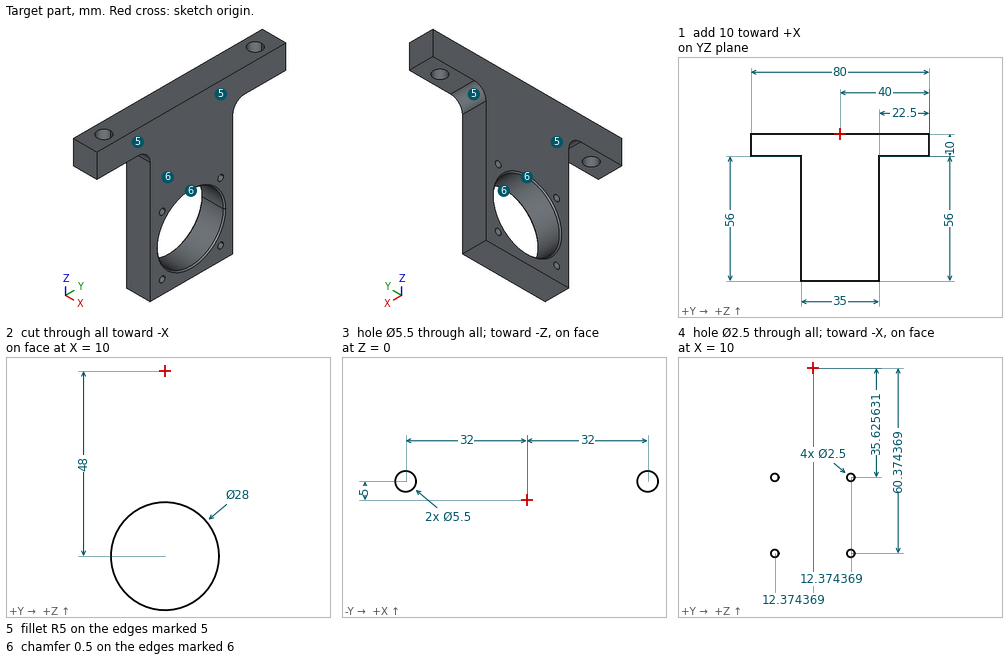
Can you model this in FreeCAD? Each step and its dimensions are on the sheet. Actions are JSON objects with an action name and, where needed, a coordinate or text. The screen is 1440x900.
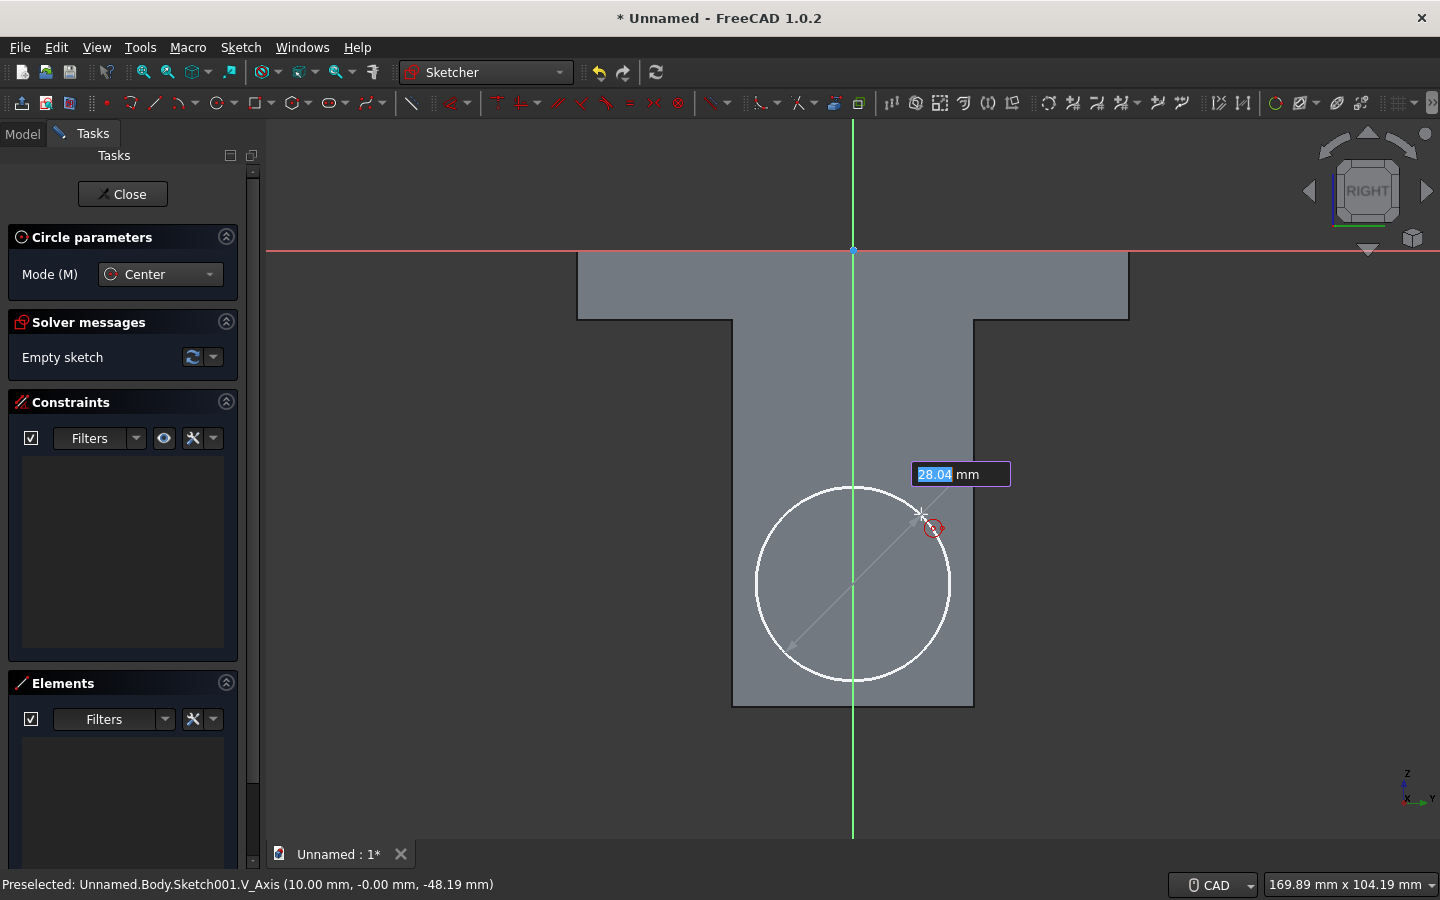
{"action": "type", "text": "28"}
{"action": "key", "text": "Return"}
{"action": "key", "text": "Escape"}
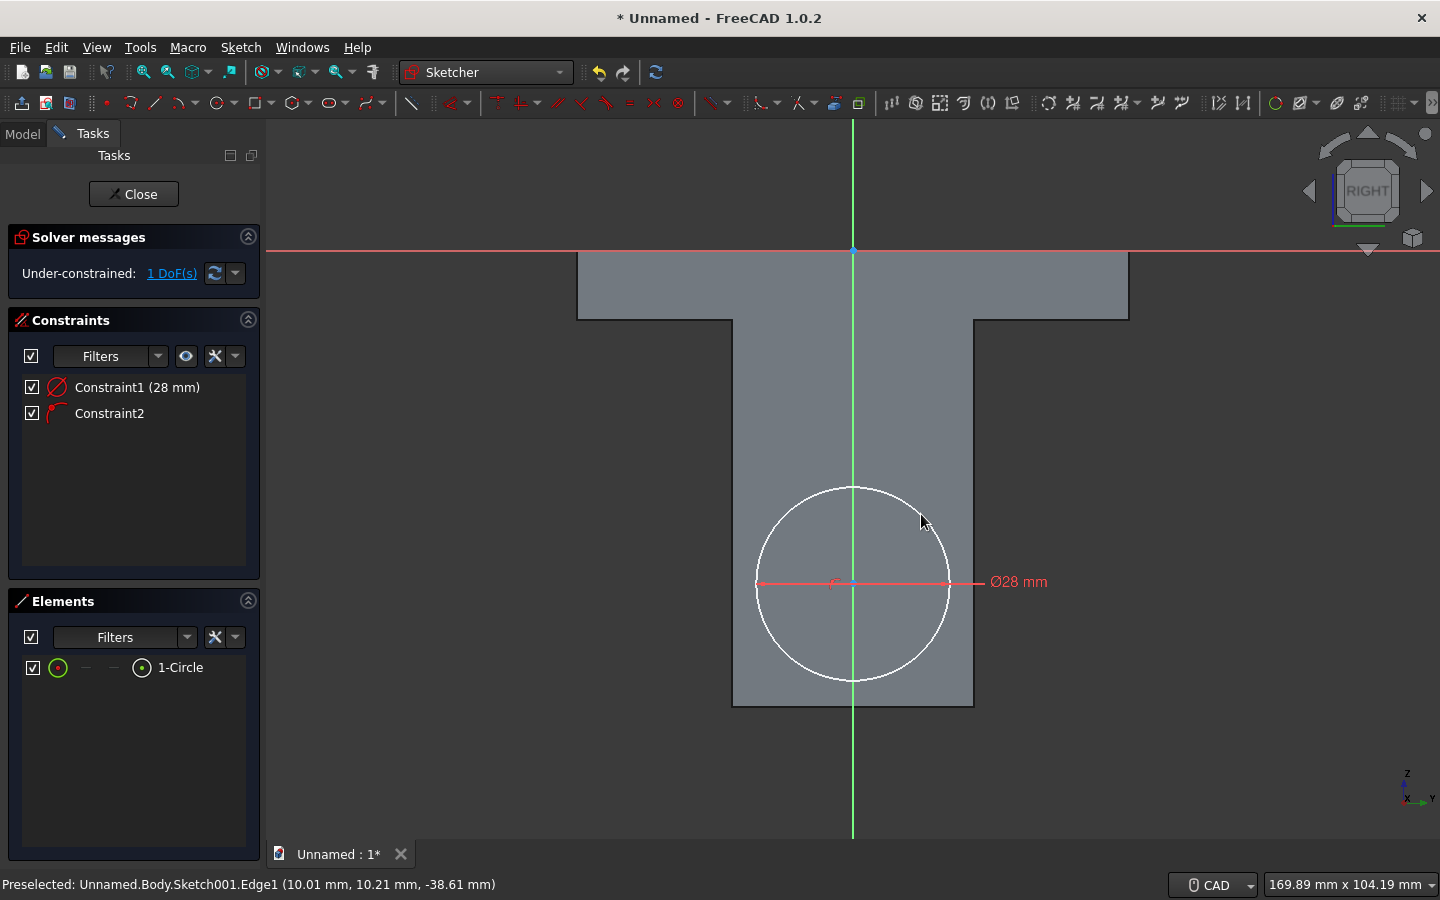
{"action": "left_click", "coordinate": [450, 104]}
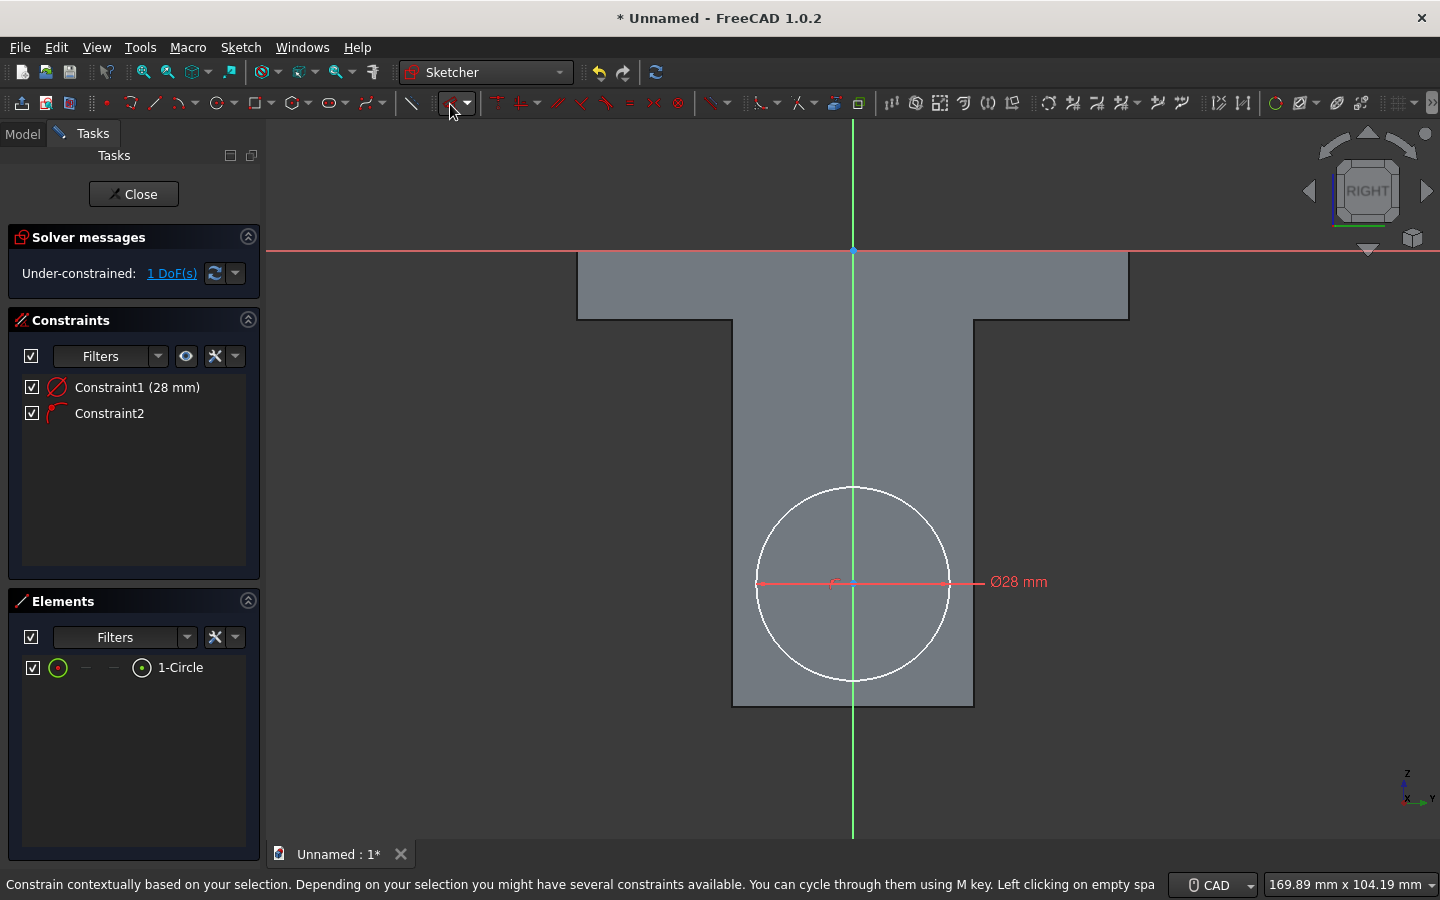
{"action": "left_click", "coordinate": [853, 584]}
{"action": "left_click", "coordinate": [887, 417]}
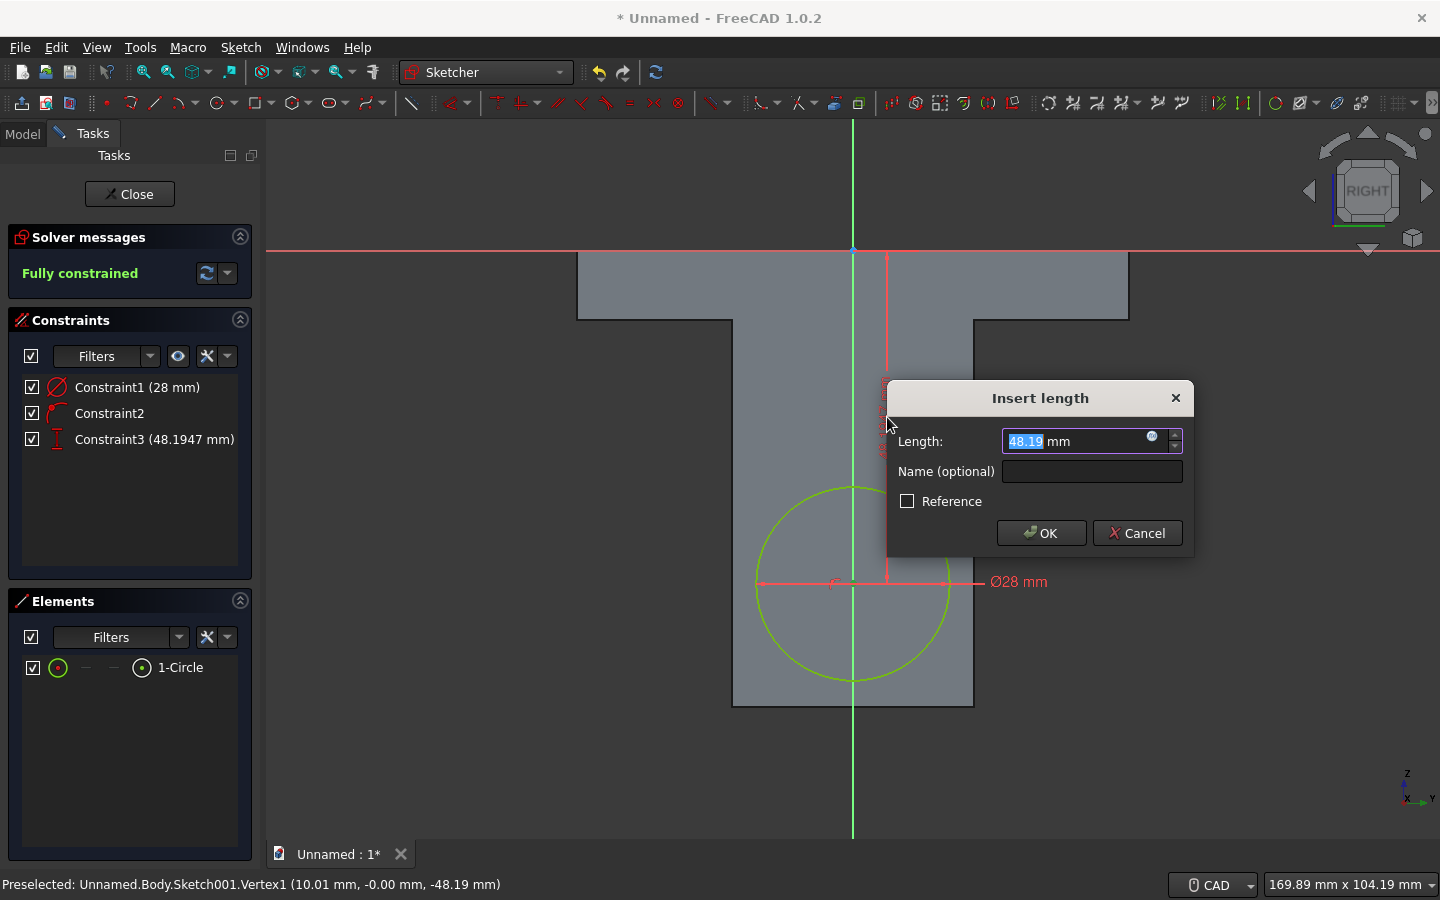
{"action": "type", "text": "48"}
{"action": "key", "text": "Return"}
{"action": "key", "text": "Escape"}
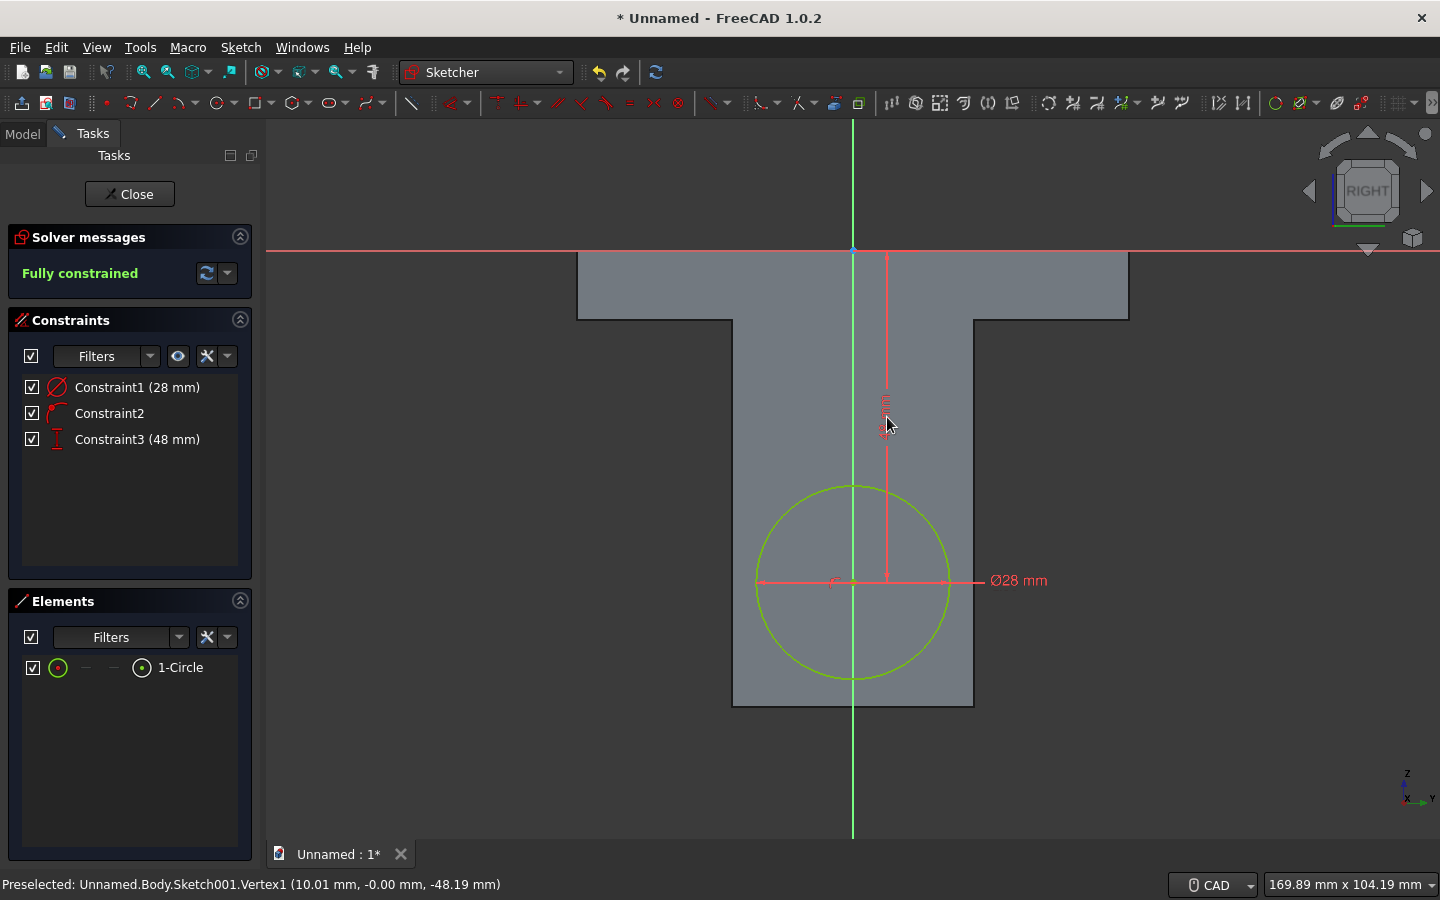
{"action": "left_click", "coordinate": [130, 194]}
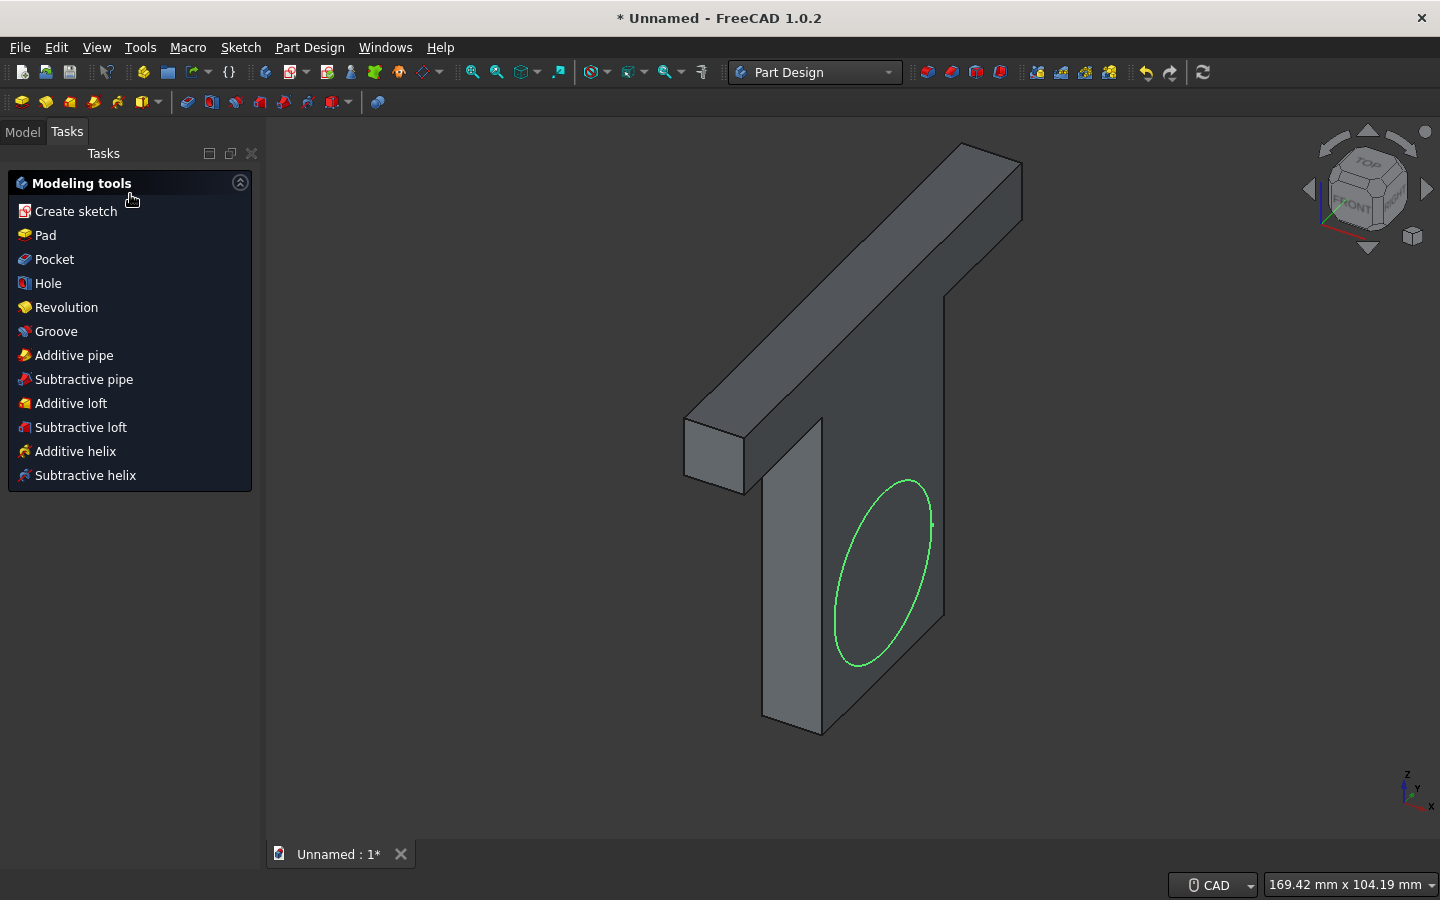
{"action": "left_click", "coordinate": [188, 102]}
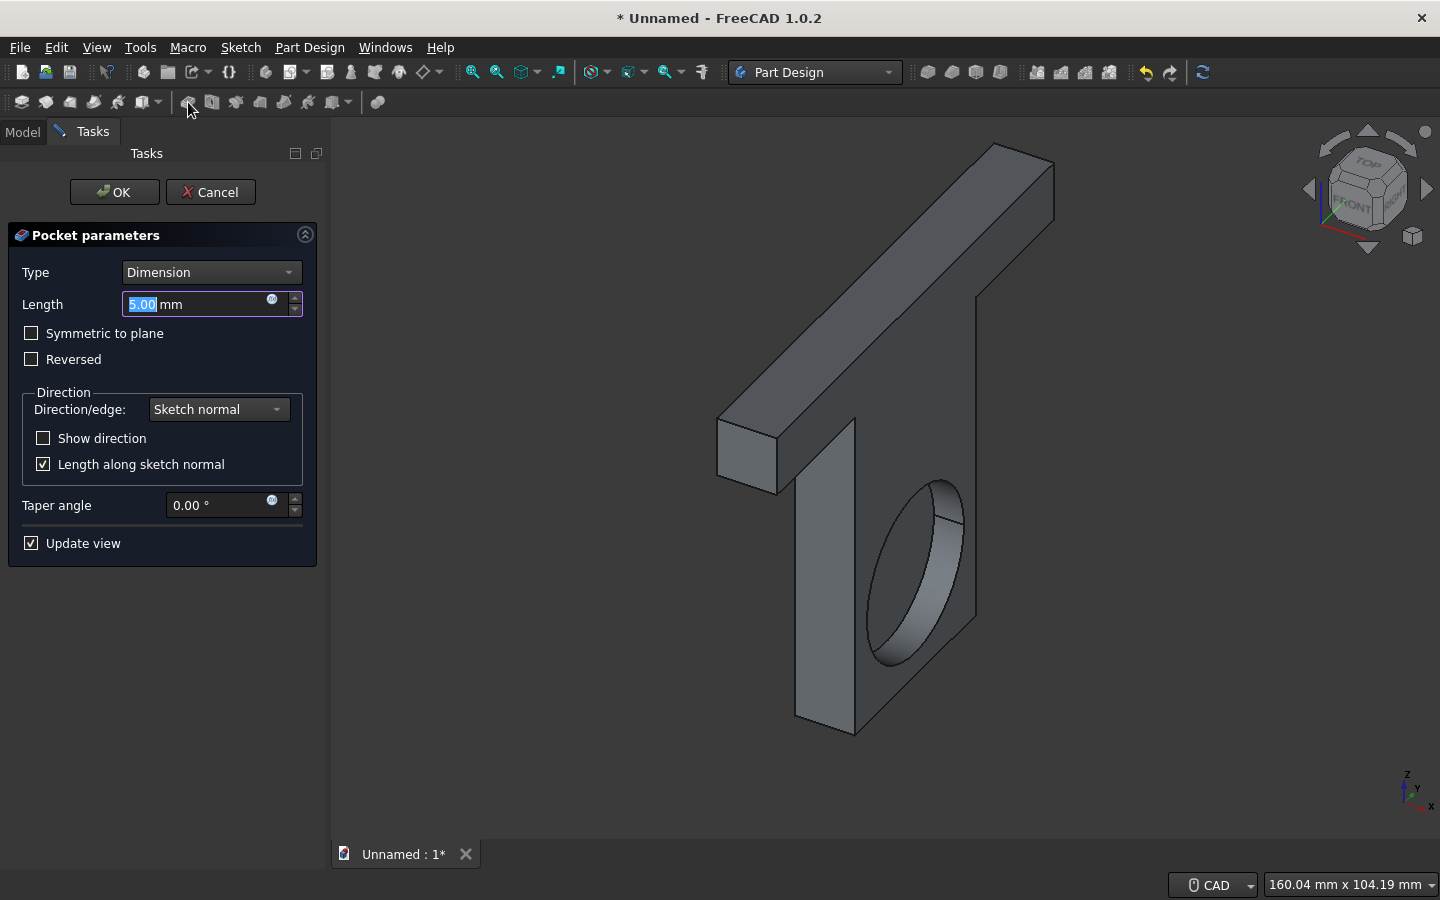
{"action": "left_click", "coordinate": [212, 272]}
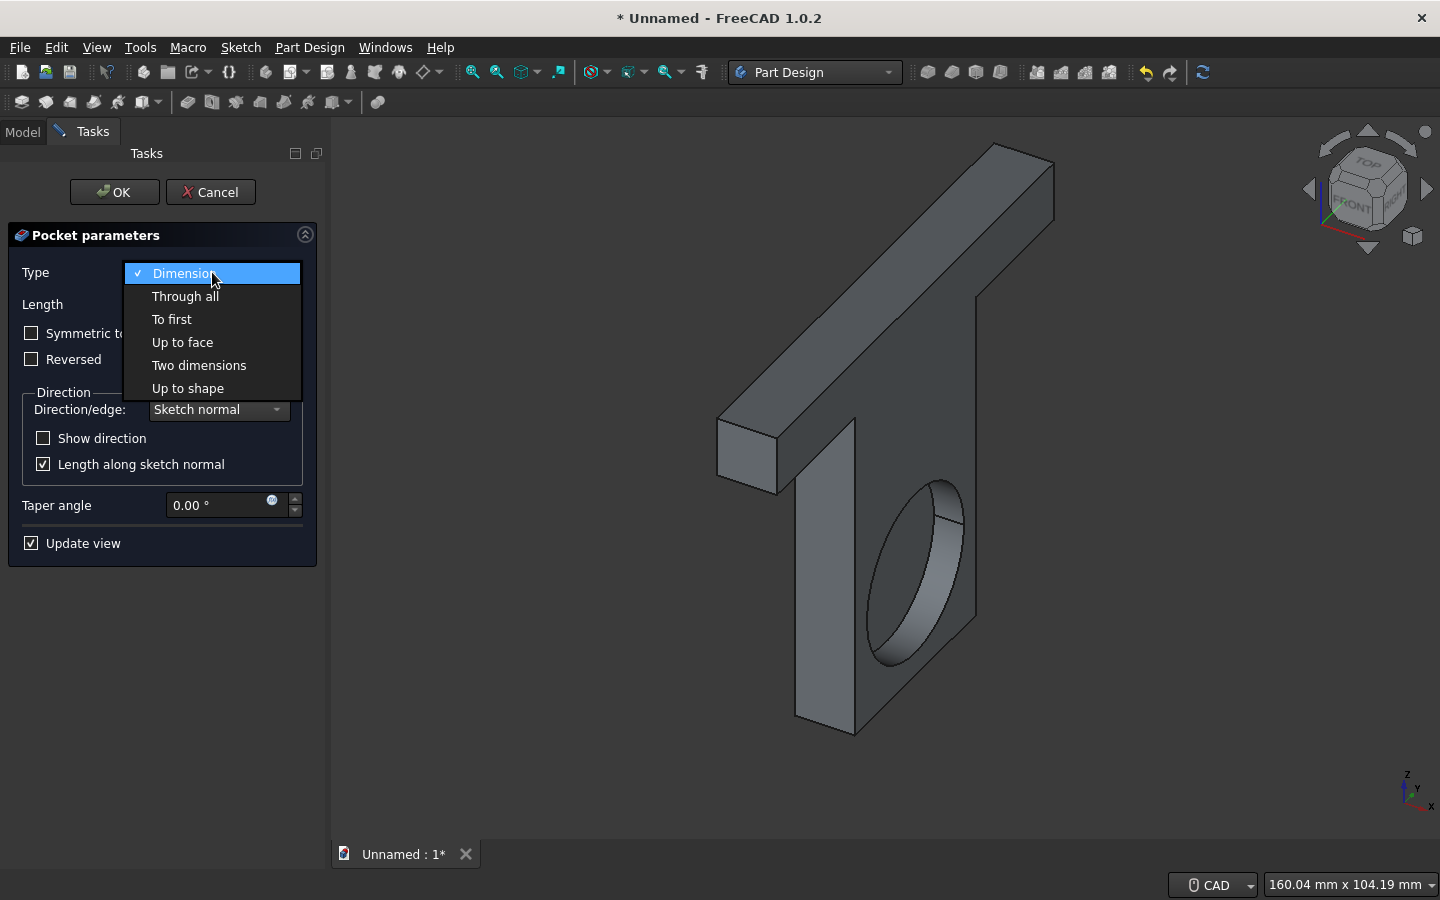
{"action": "left_click", "coordinate": [212, 296]}